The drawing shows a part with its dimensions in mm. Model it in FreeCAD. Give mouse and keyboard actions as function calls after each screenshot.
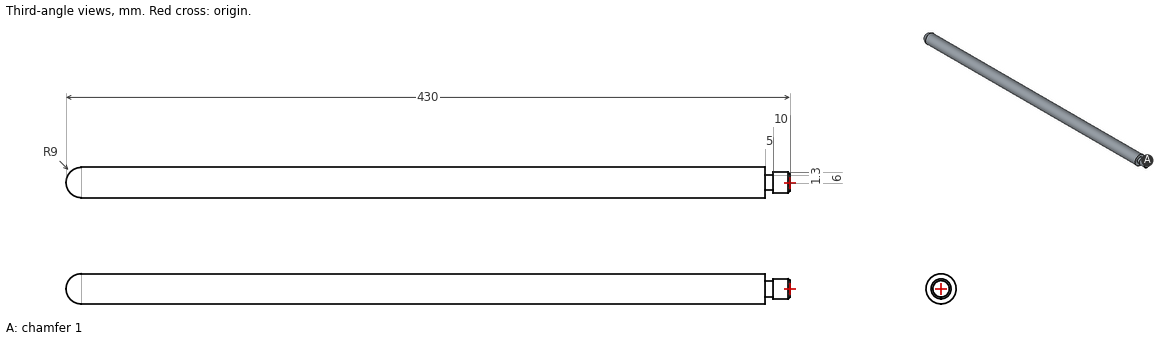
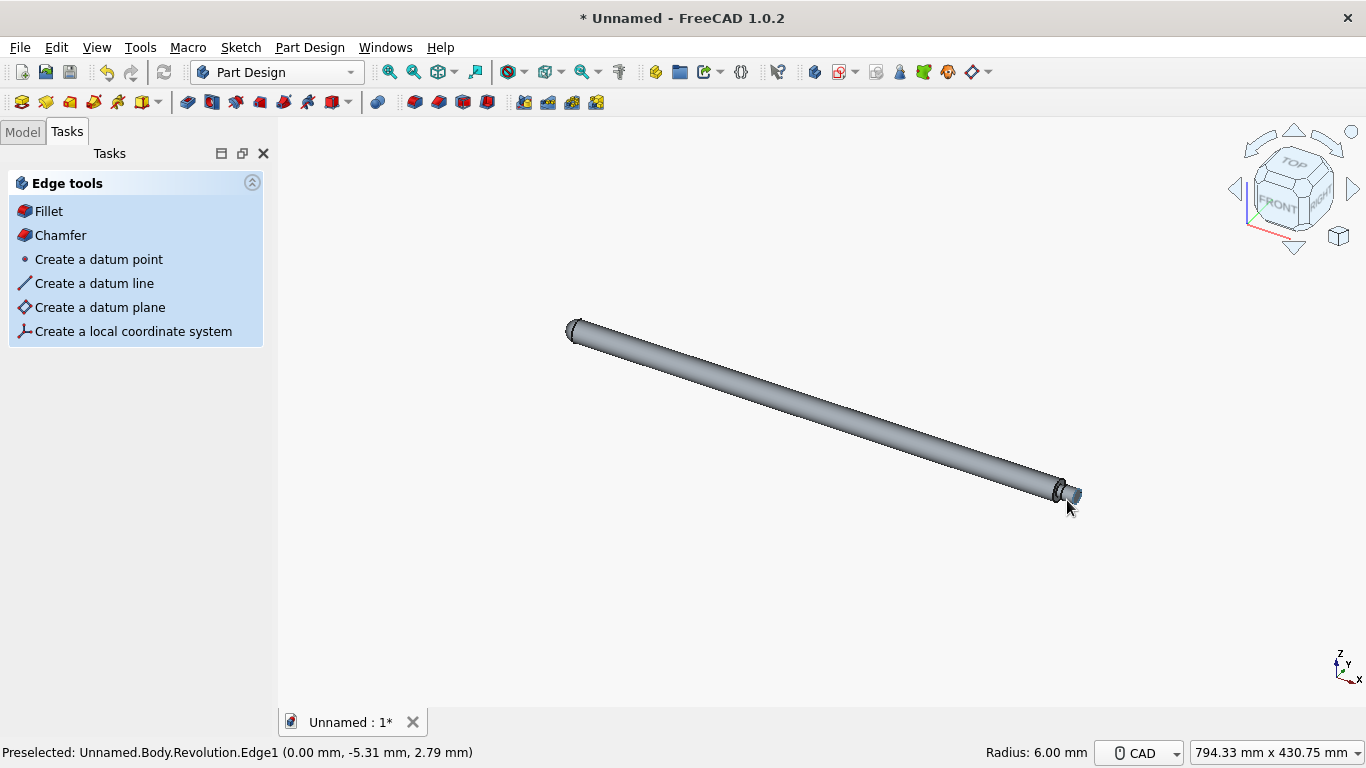
click(440, 102)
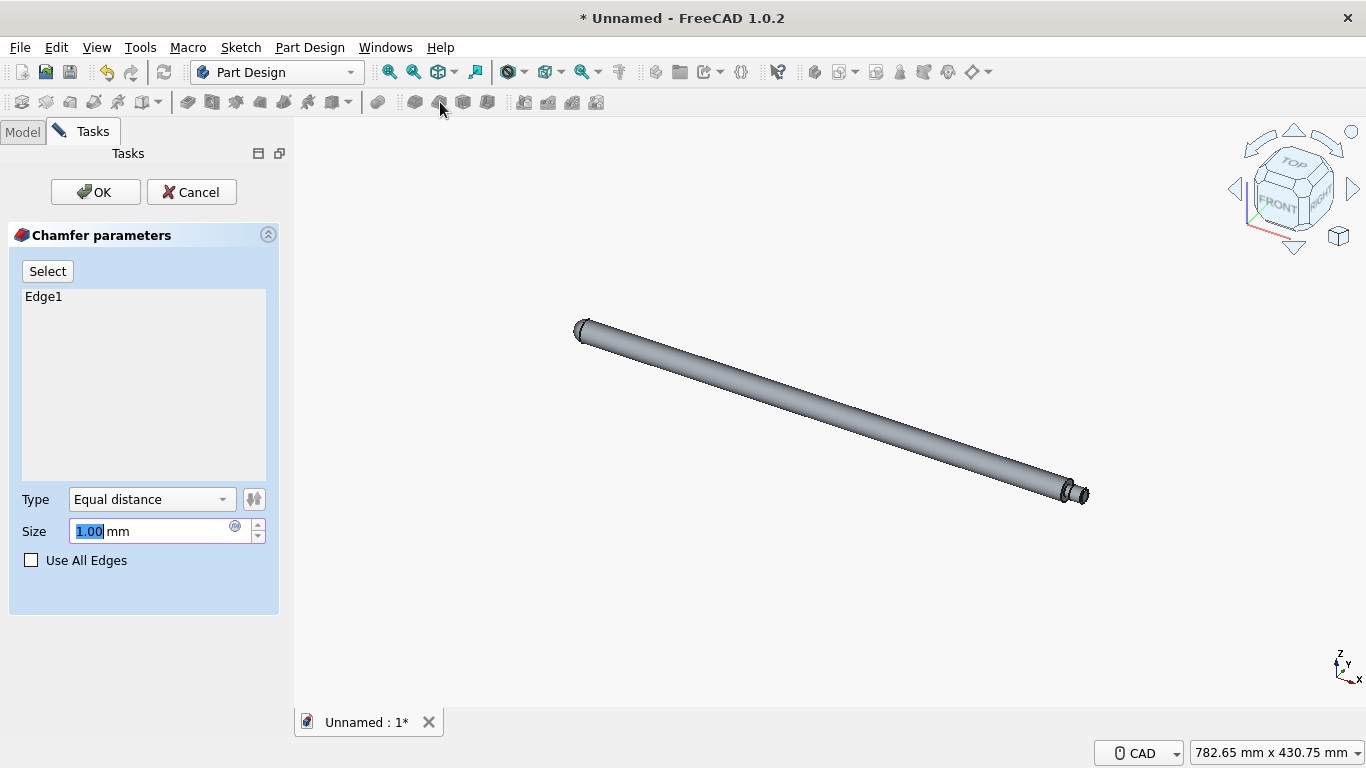
text(1)
key(Tab)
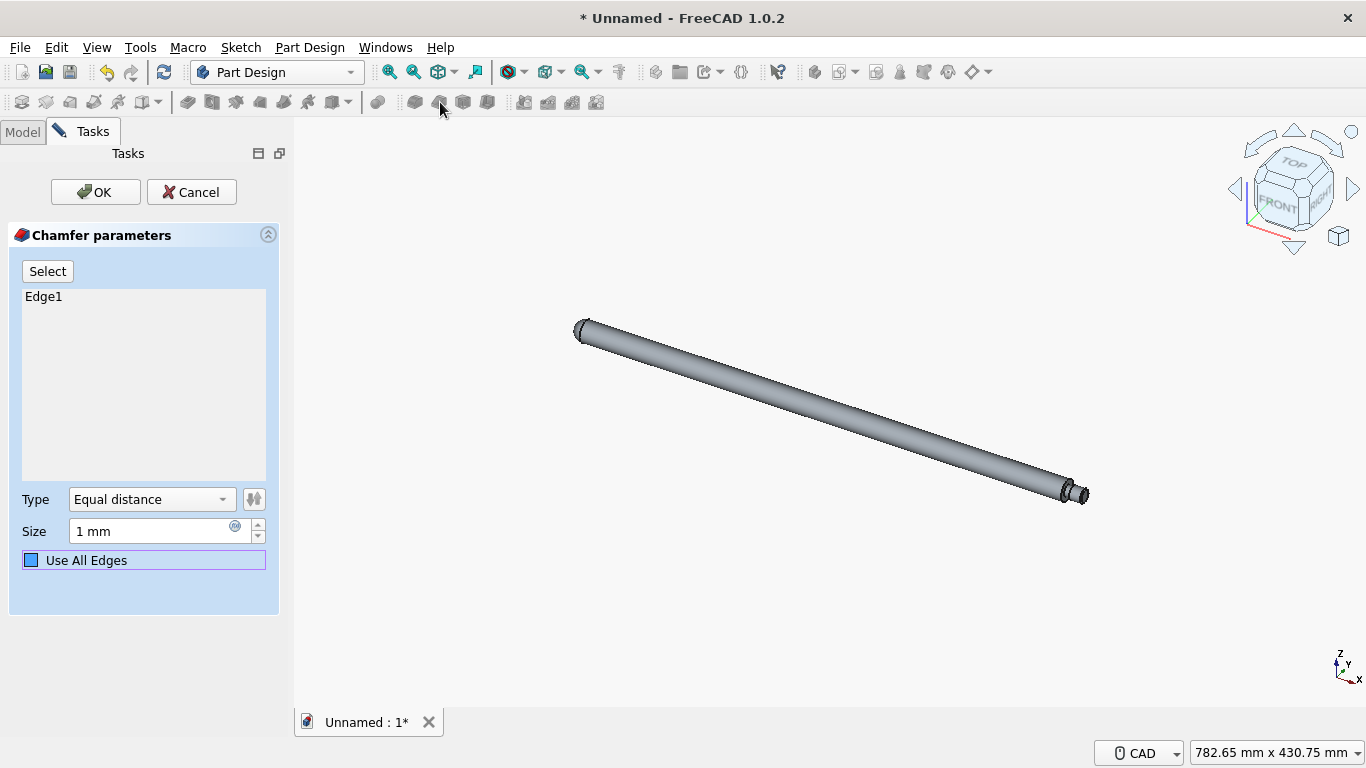
click(96, 192)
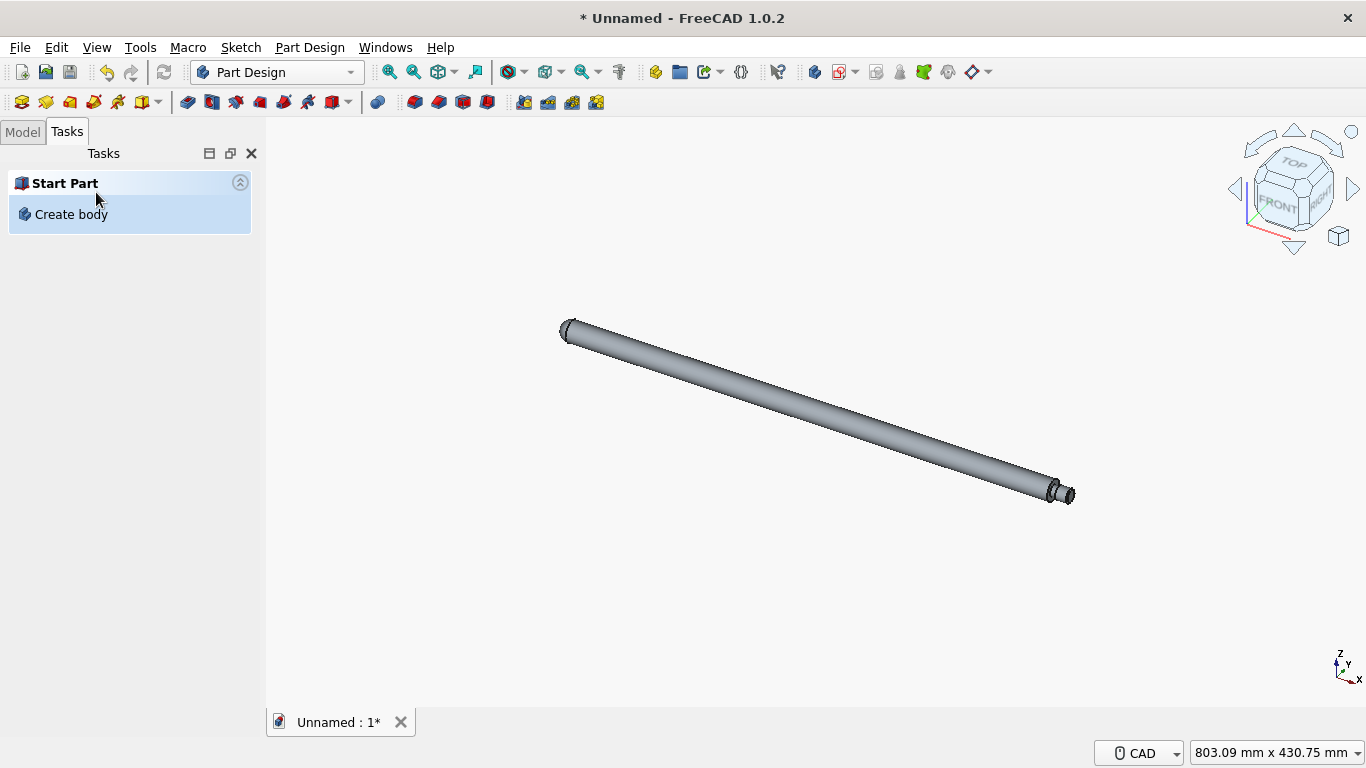
key(0)